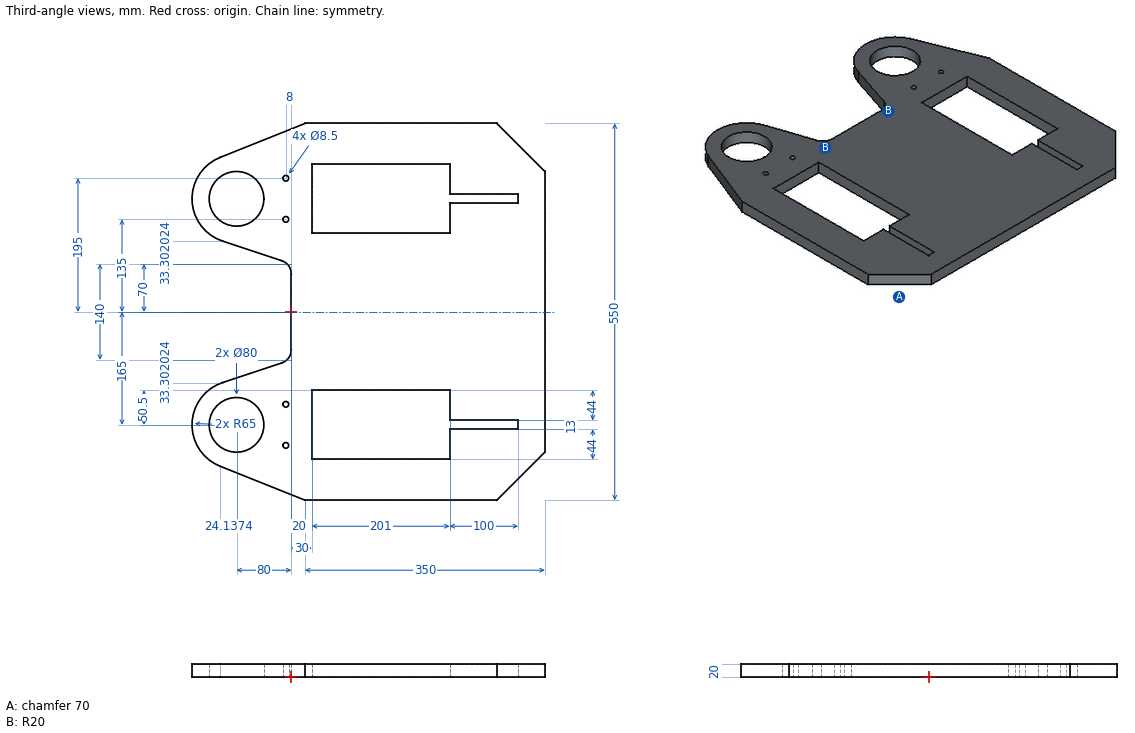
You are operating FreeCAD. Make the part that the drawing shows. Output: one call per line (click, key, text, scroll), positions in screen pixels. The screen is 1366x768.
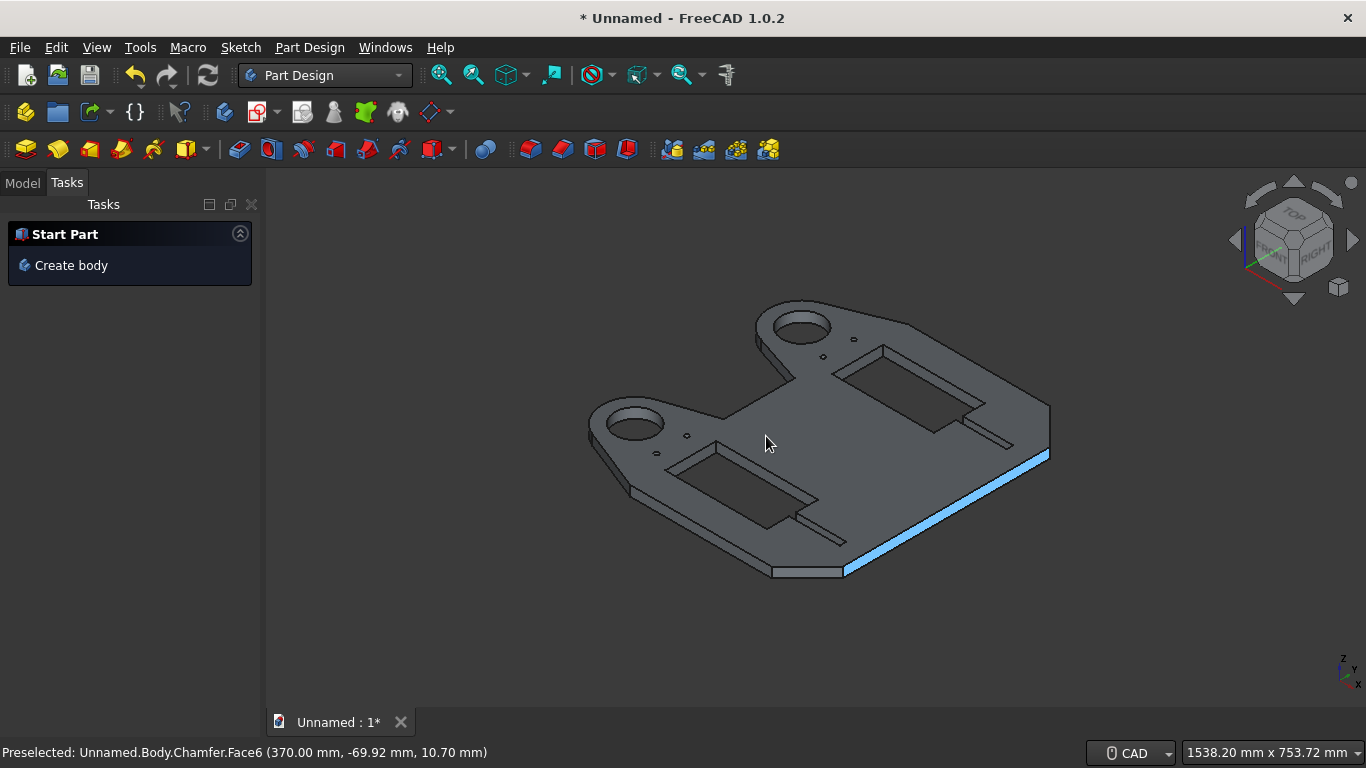
scroll(724, 424, up, 6)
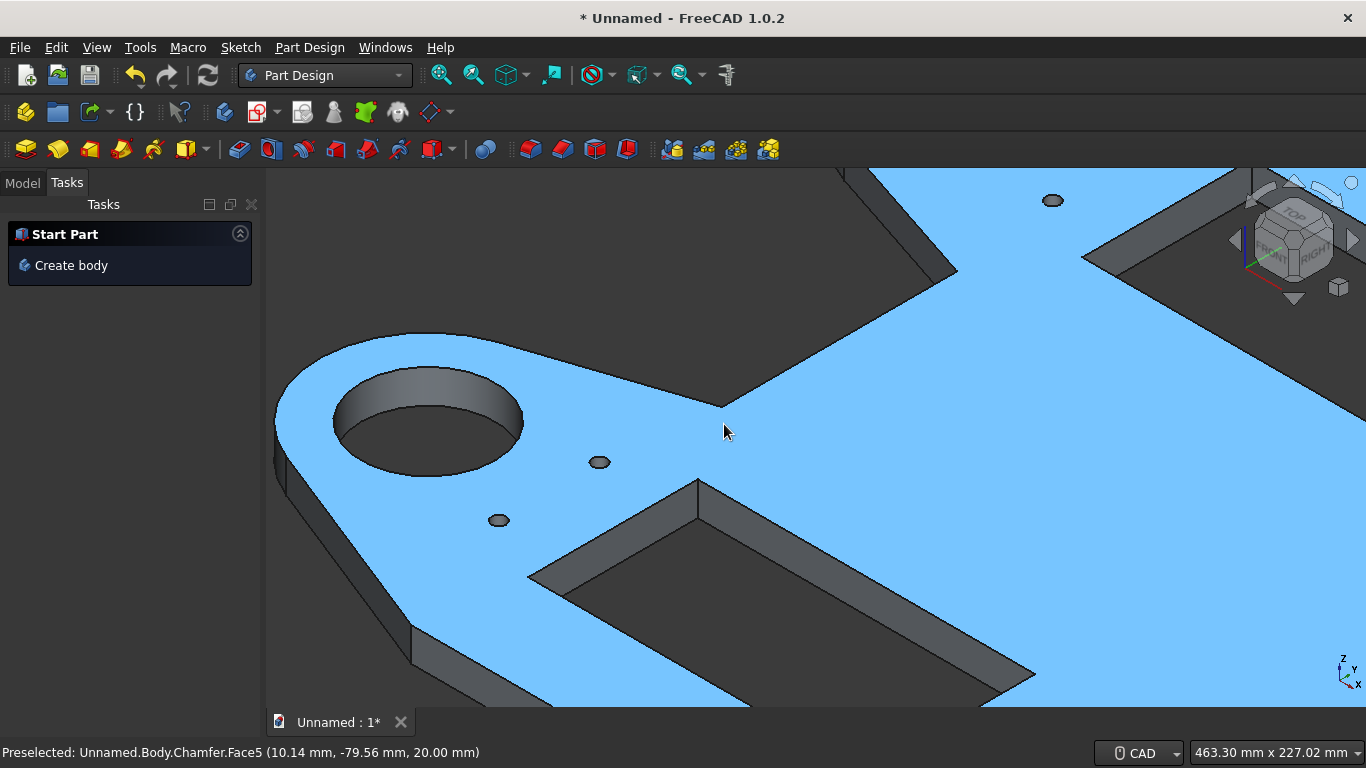
key(v)
key(f)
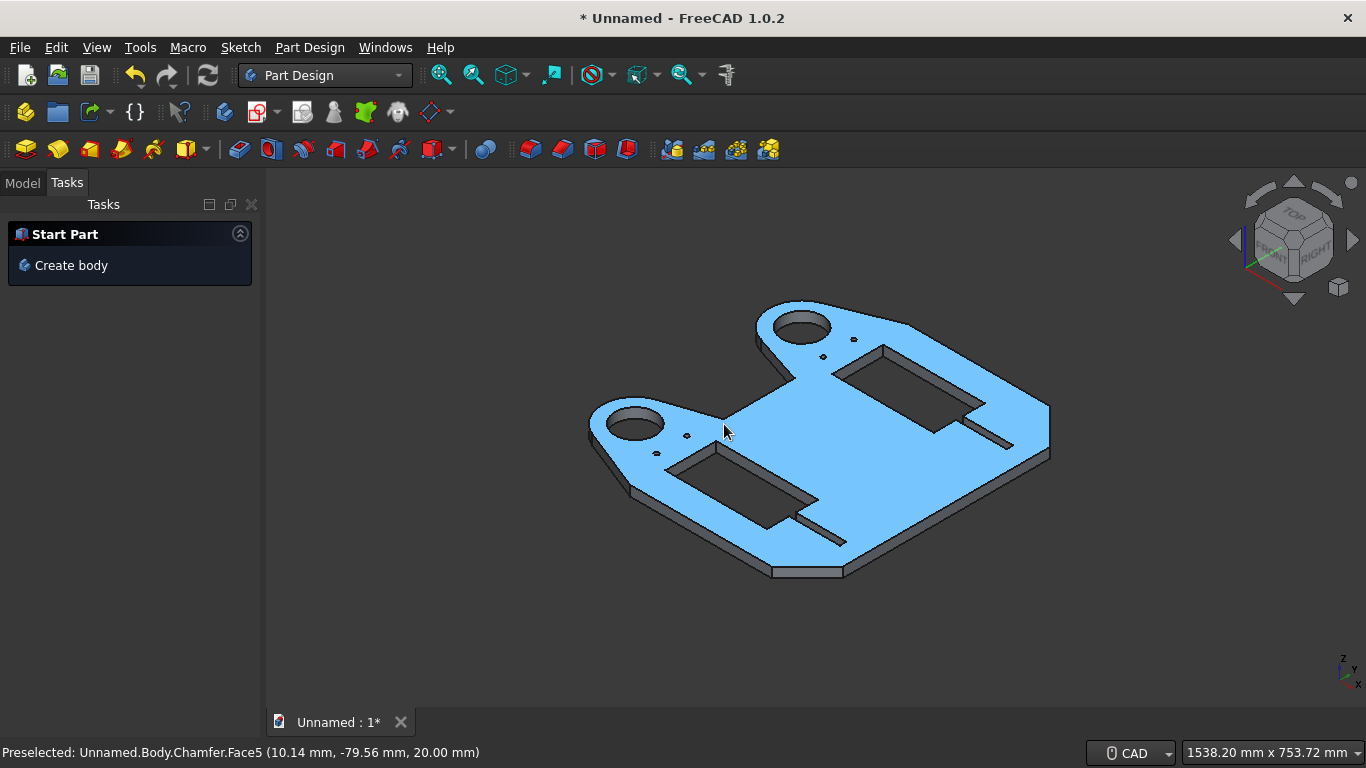
key(2)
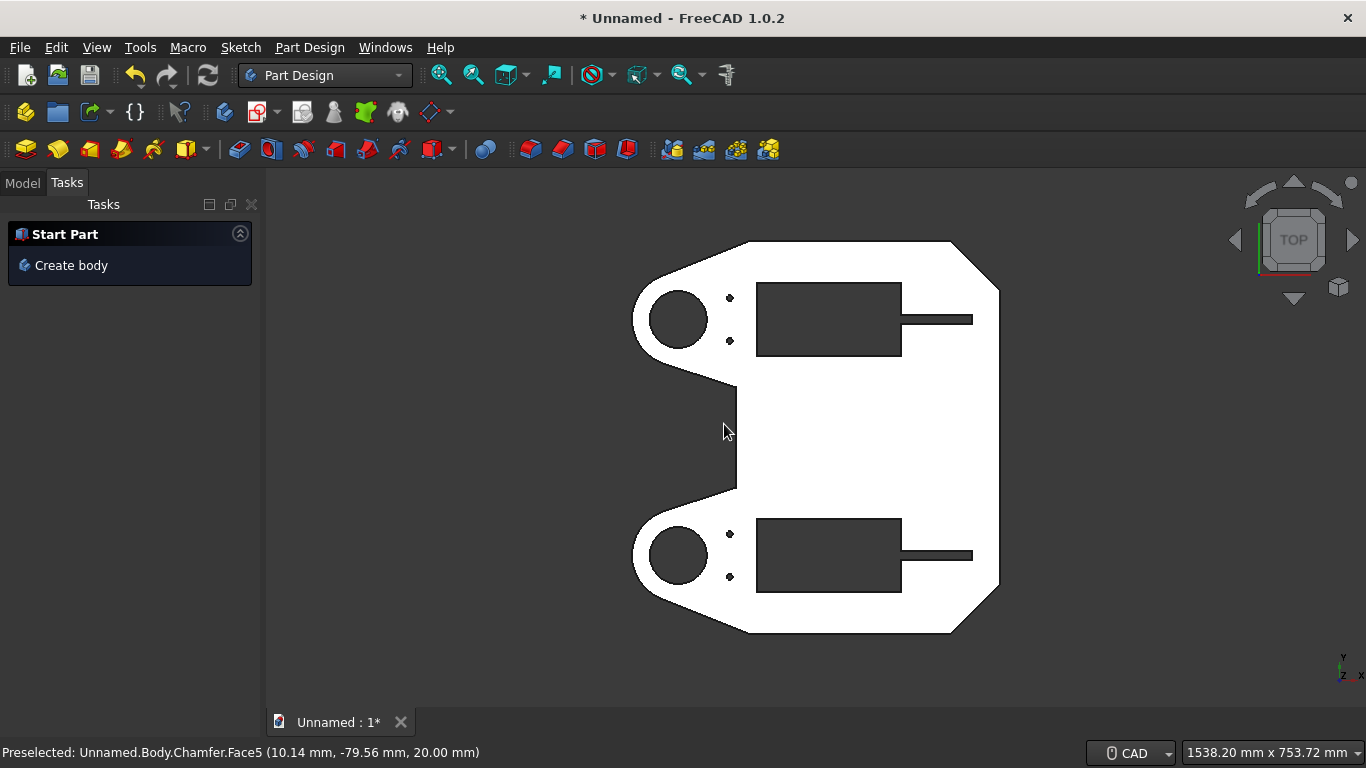
scroll(736, 487, up, 6)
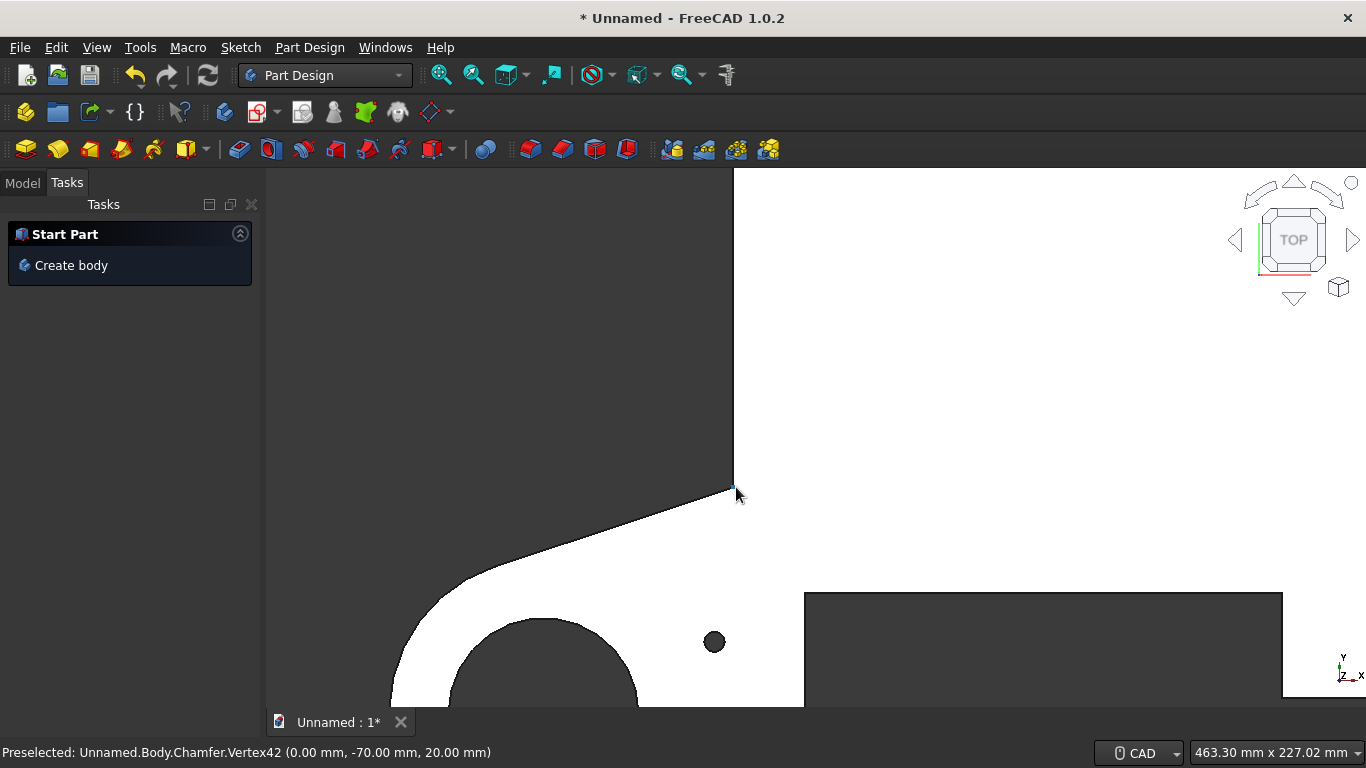
click(442, 76)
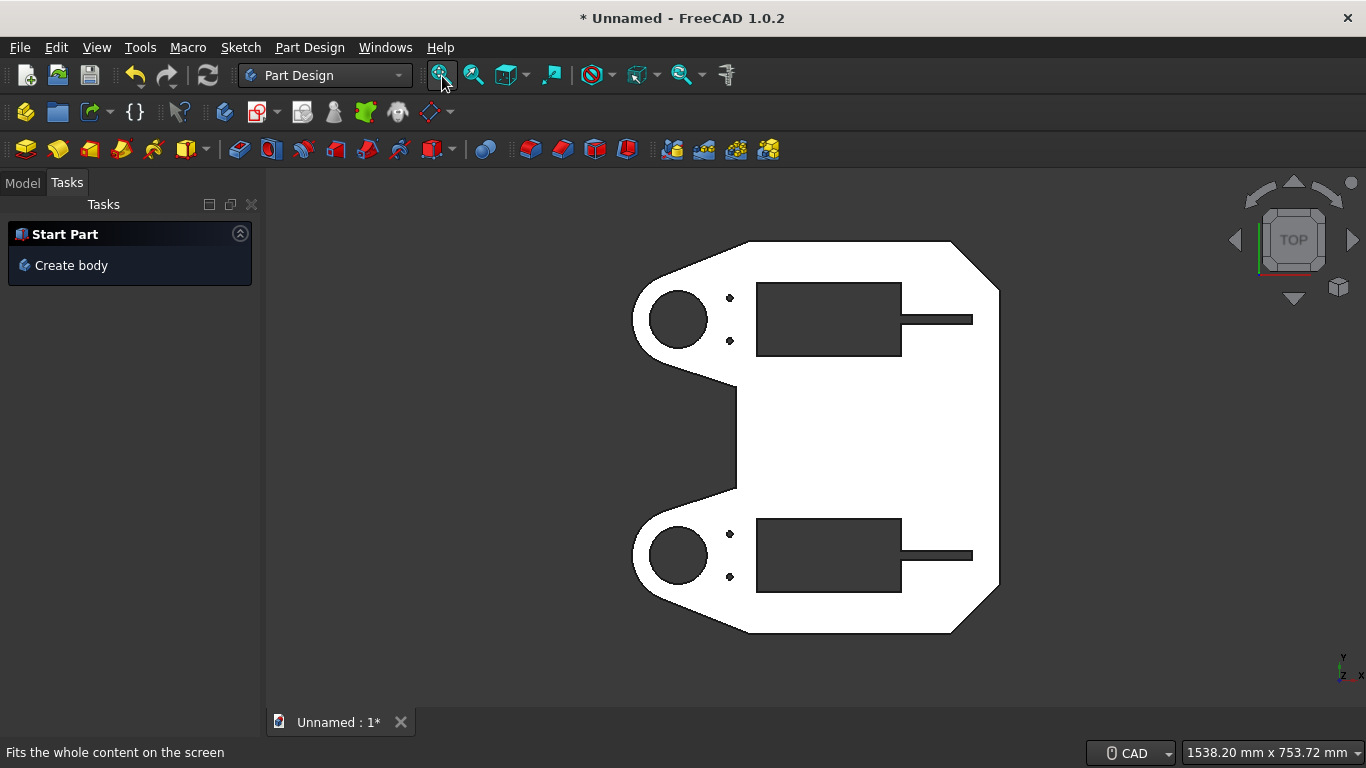
key(1)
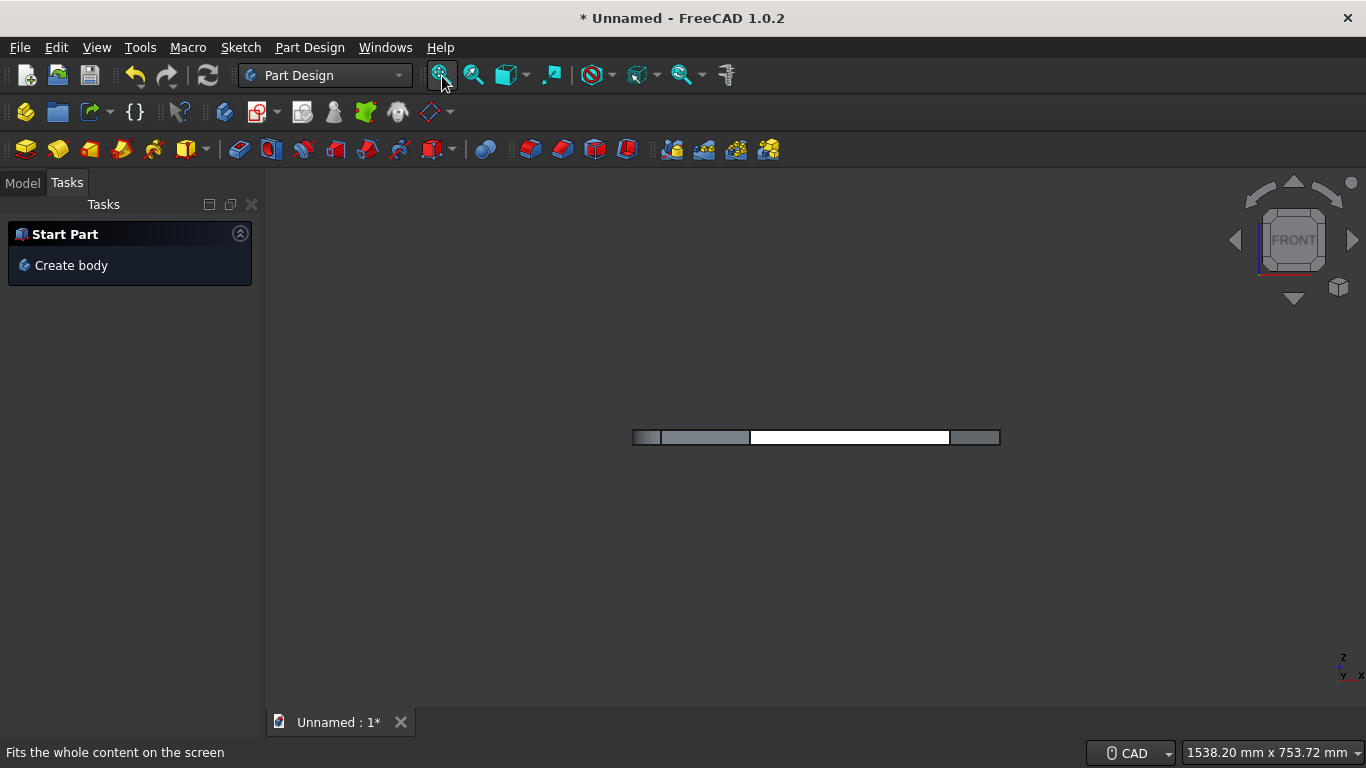
key(v)
key(f)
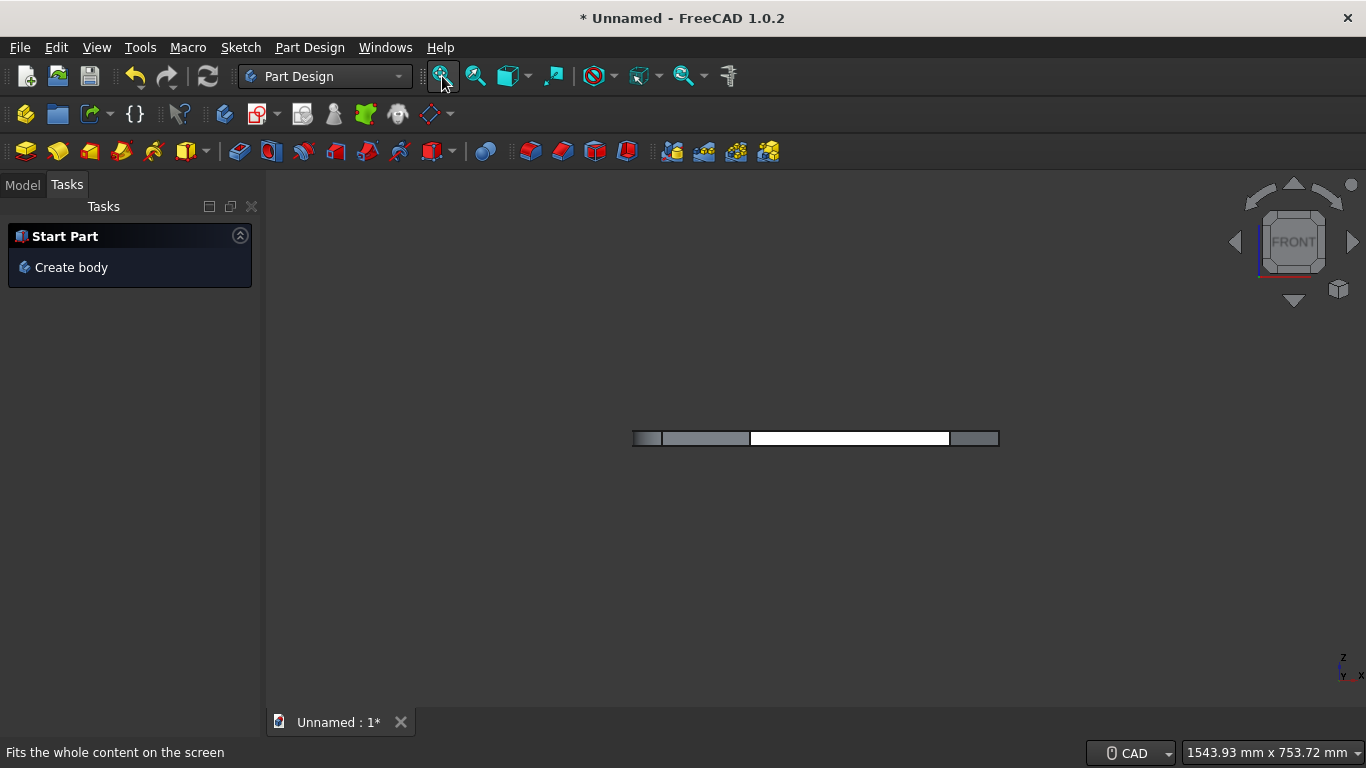
scroll(736, 438, up, 6)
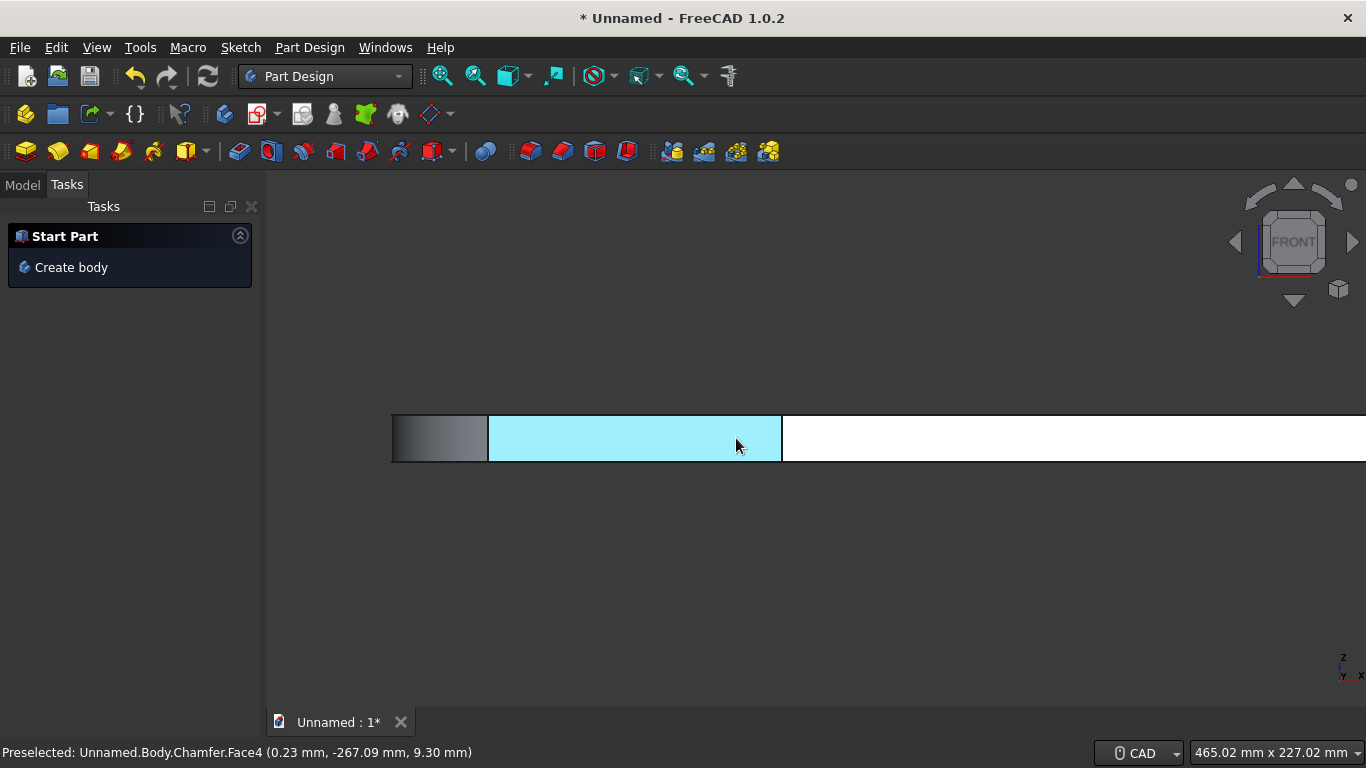
key(v)
key(f)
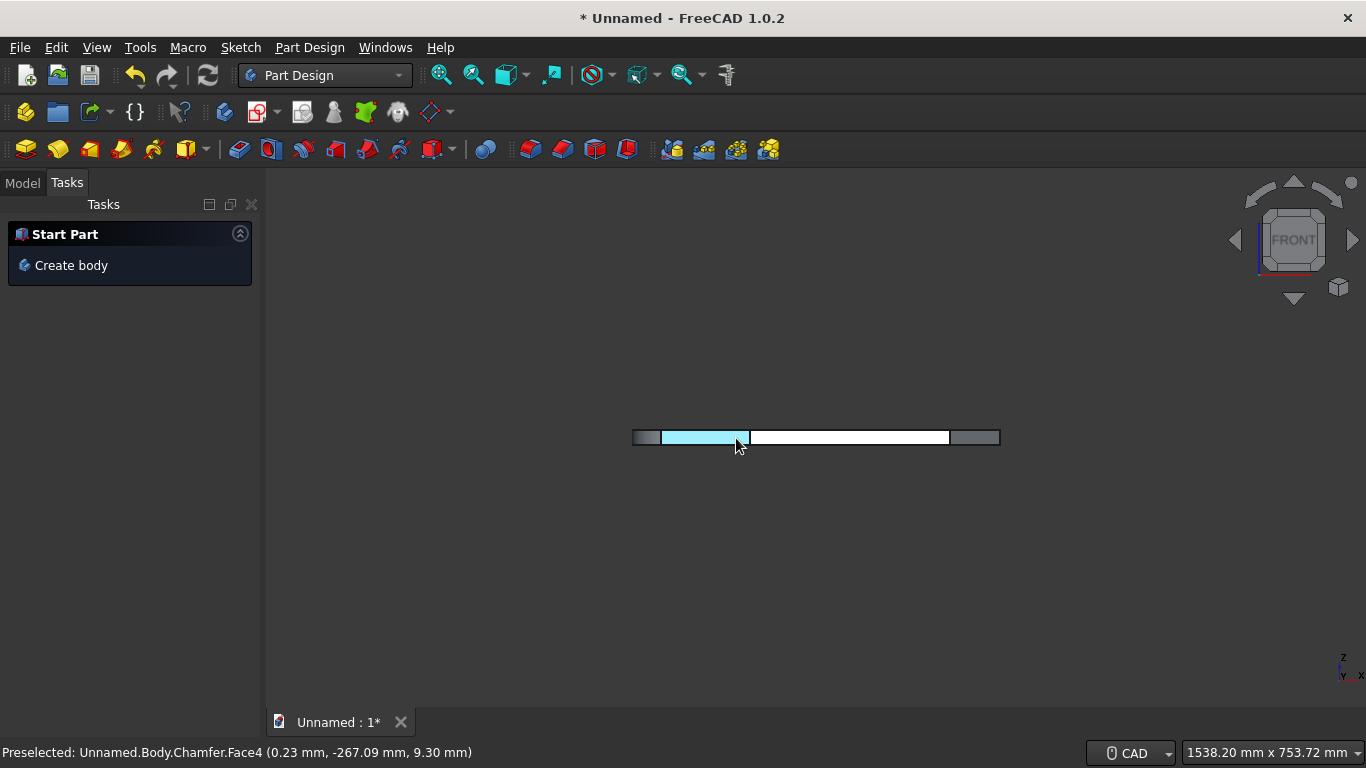
key(3)